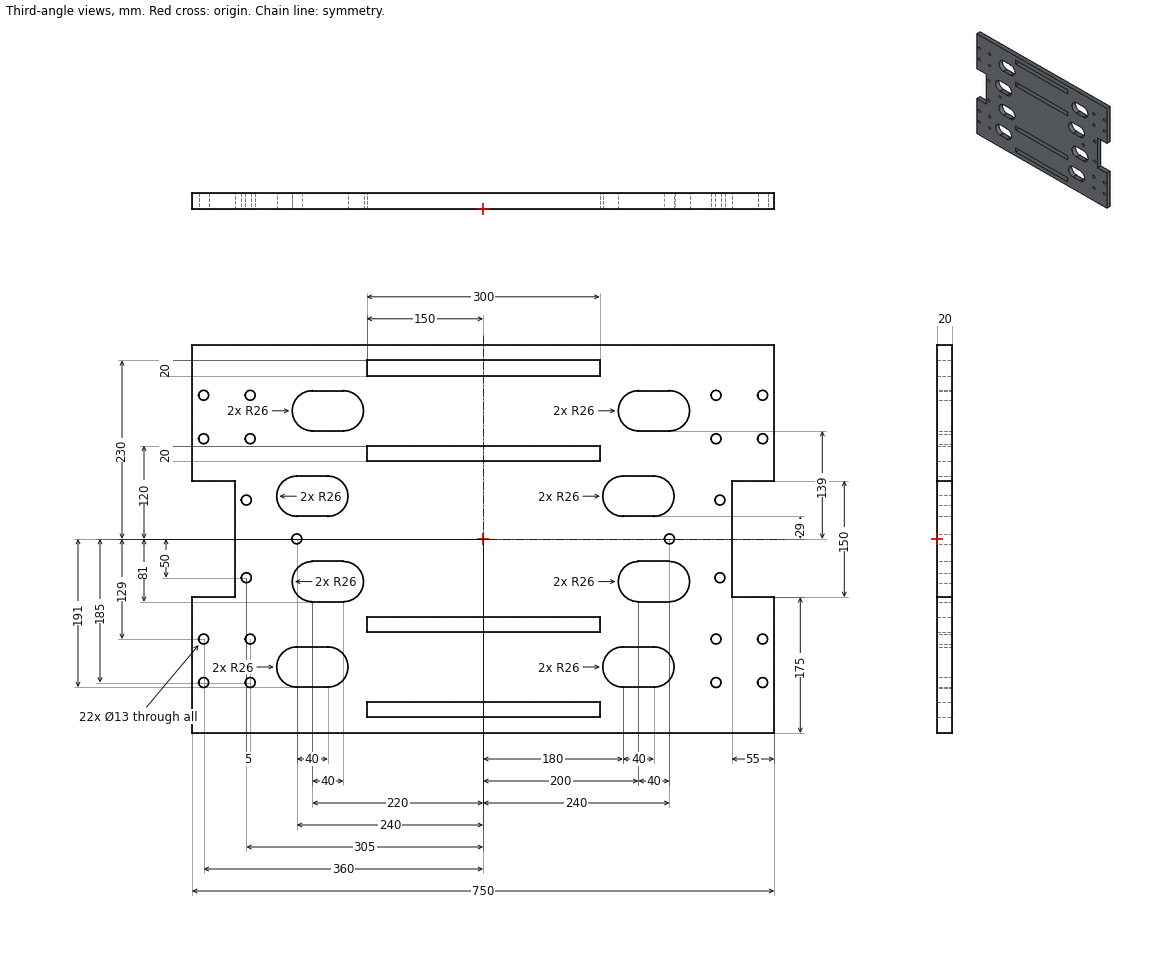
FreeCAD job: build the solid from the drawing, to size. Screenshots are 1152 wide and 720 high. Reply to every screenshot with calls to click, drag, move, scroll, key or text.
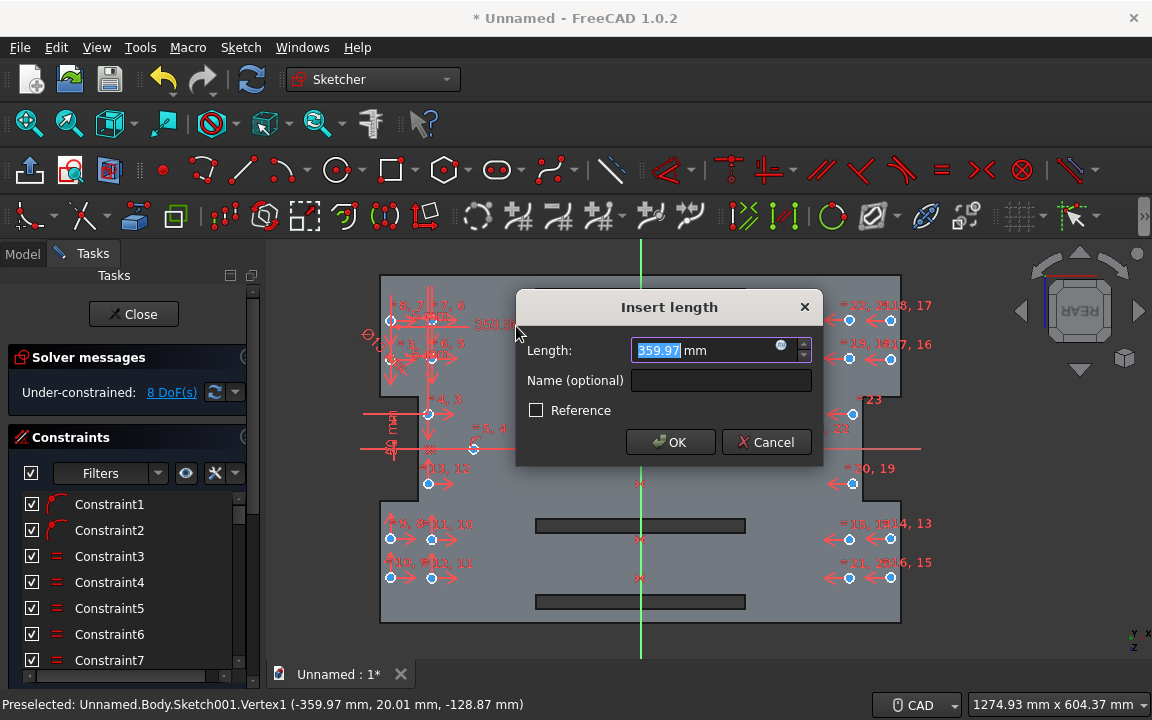
text(360)
key(Return)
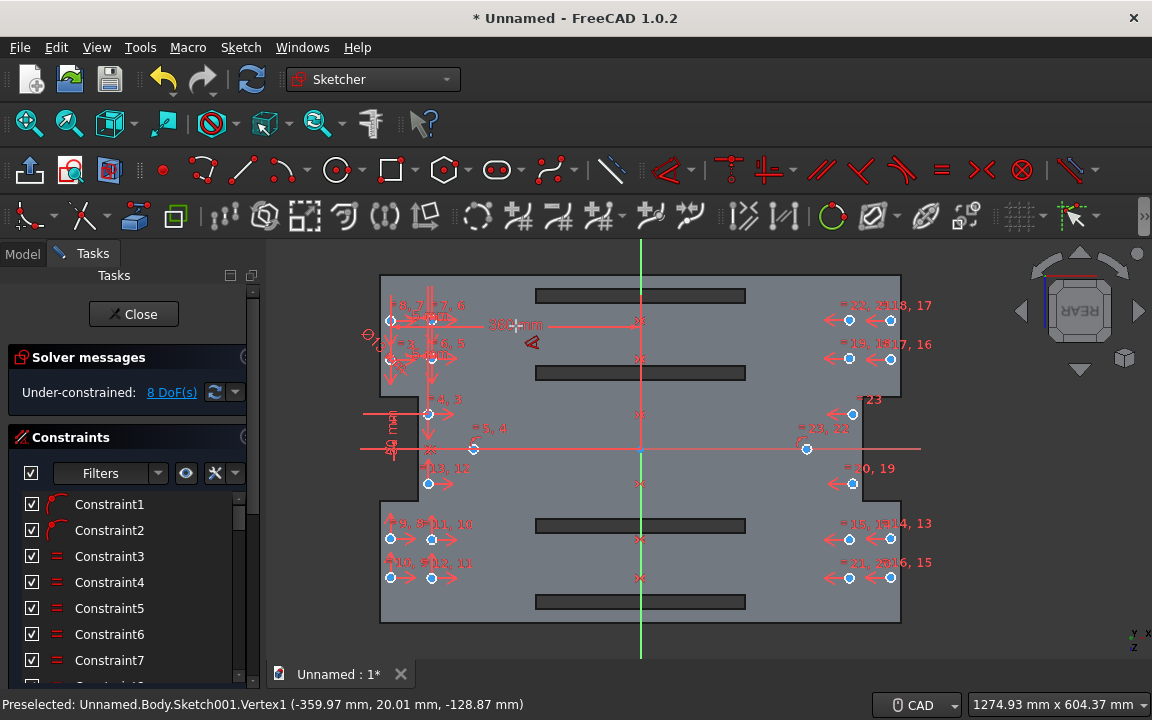
click(391, 360)
click(357, 404)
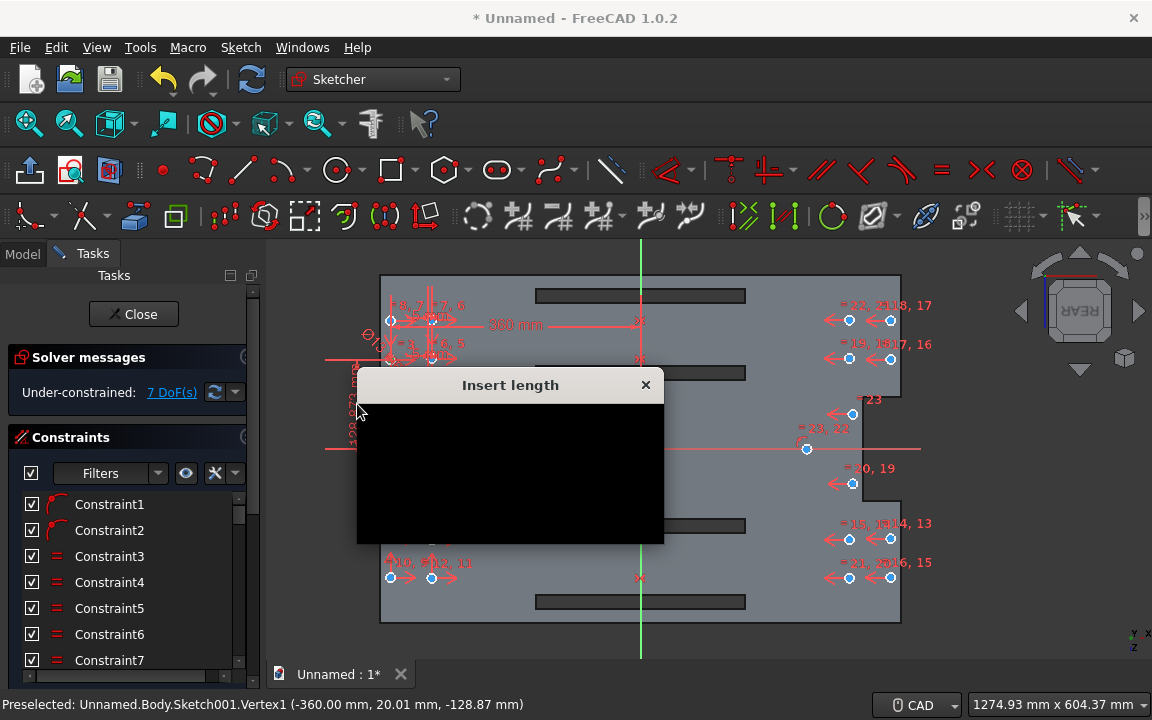
text(129)
key(Return)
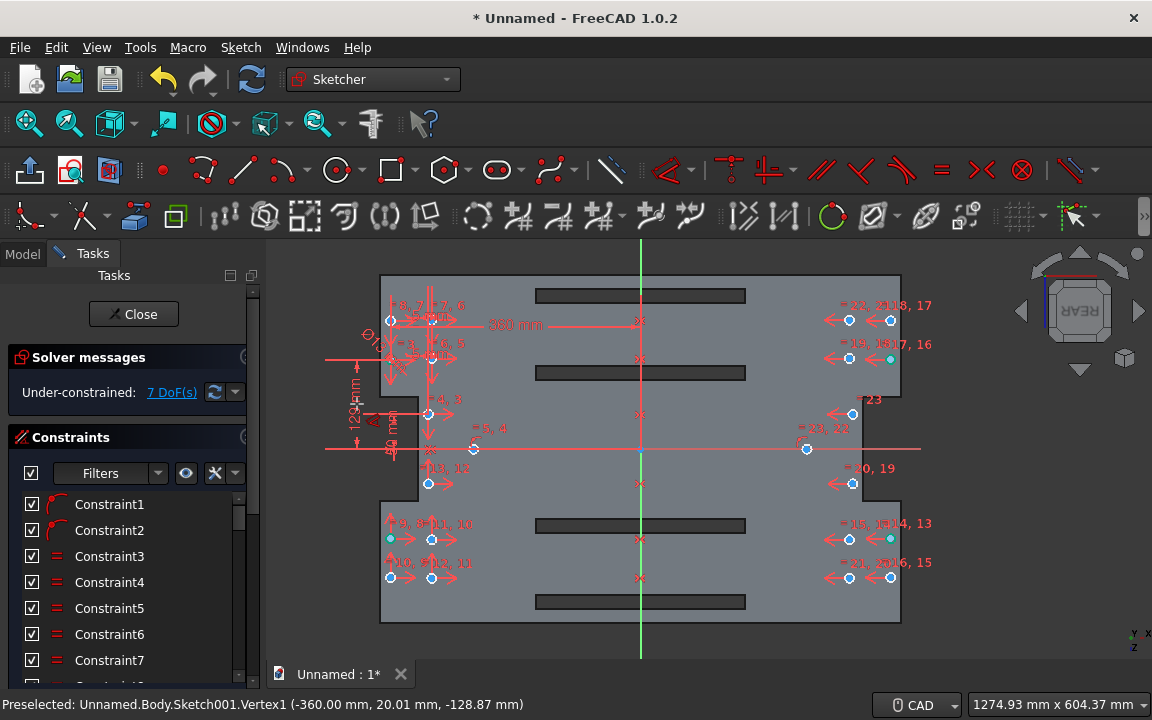
click(428, 414)
click(535, 380)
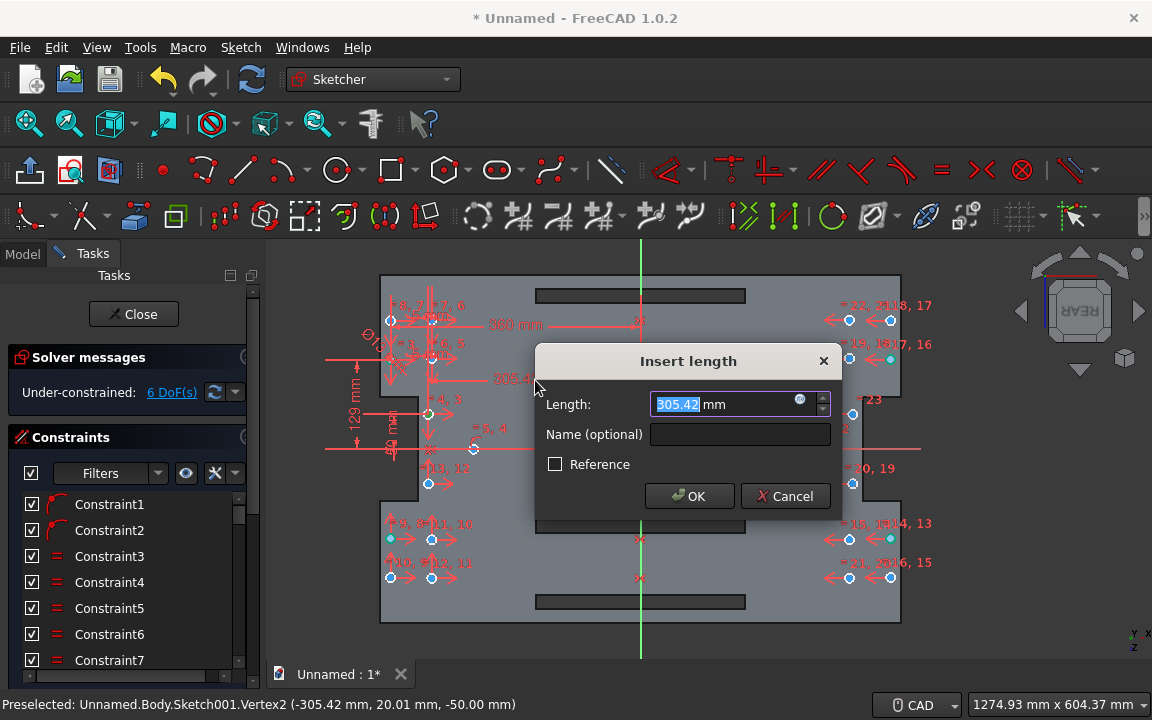
text(305)
key(Return)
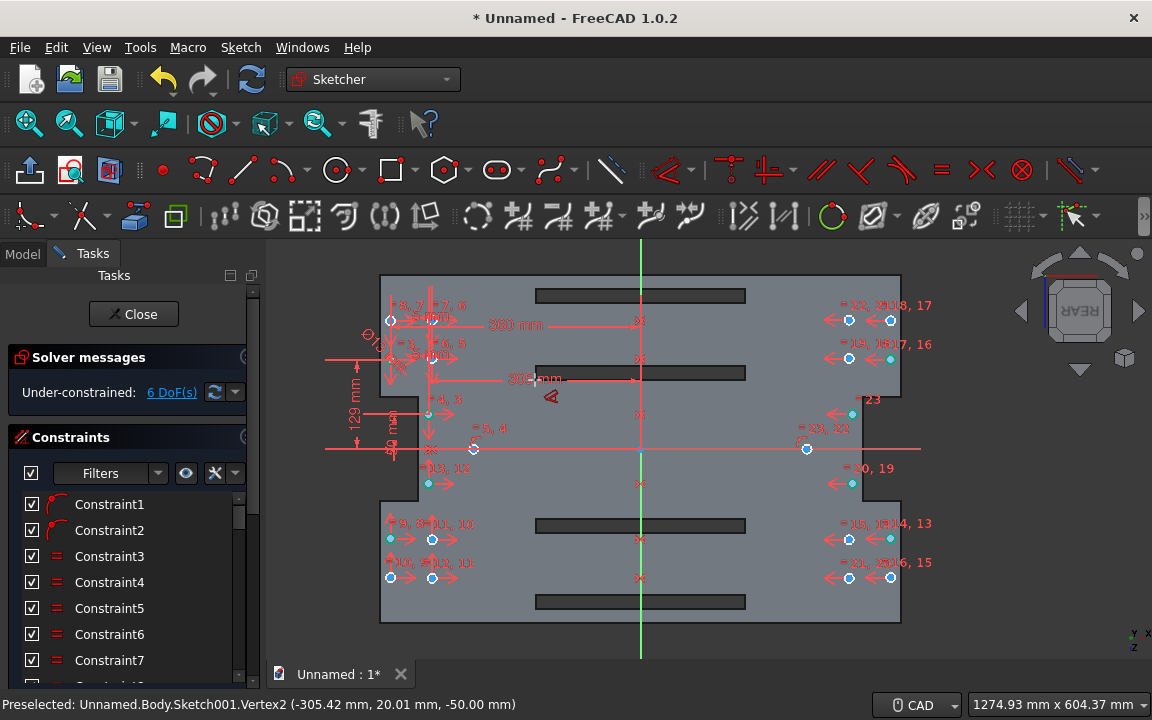
click(474, 449)
click(557, 483)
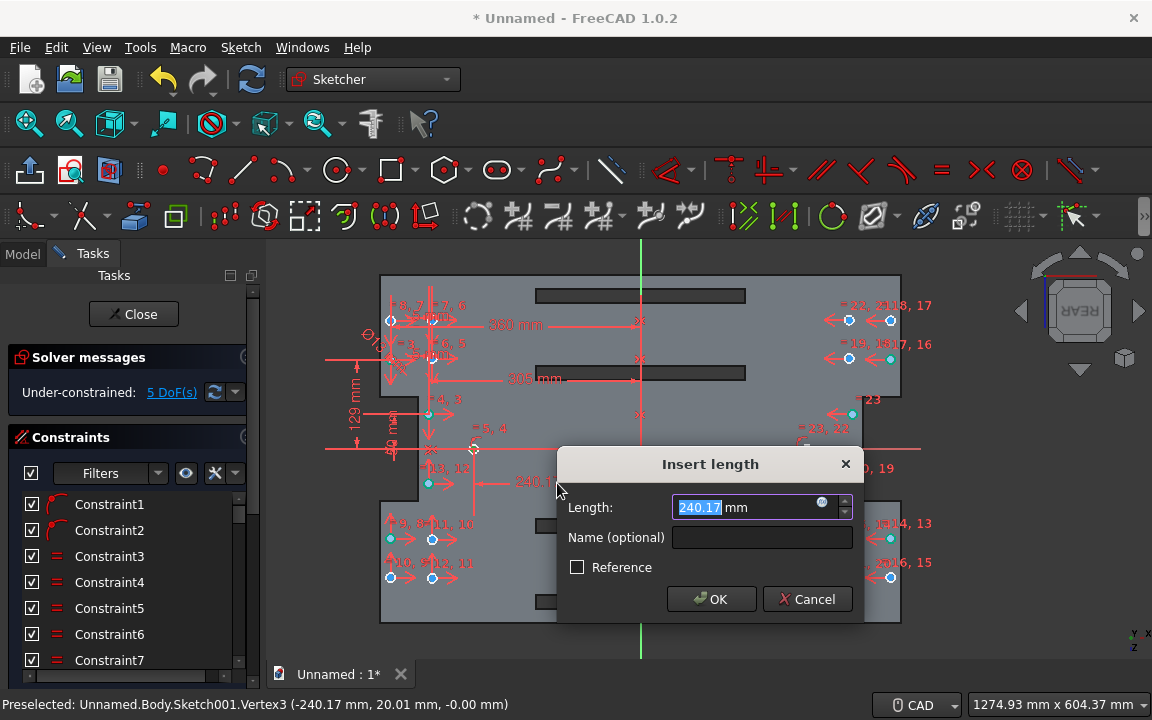
text(240)
key(Return)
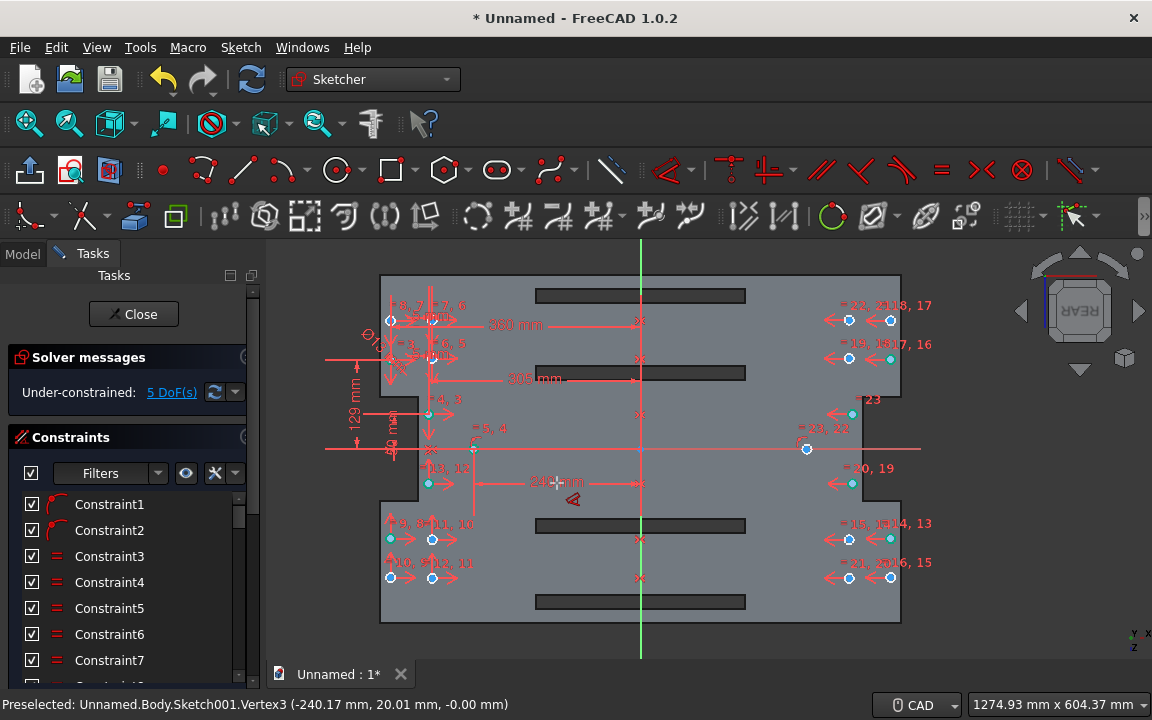
click(432, 359)
click(398, 383)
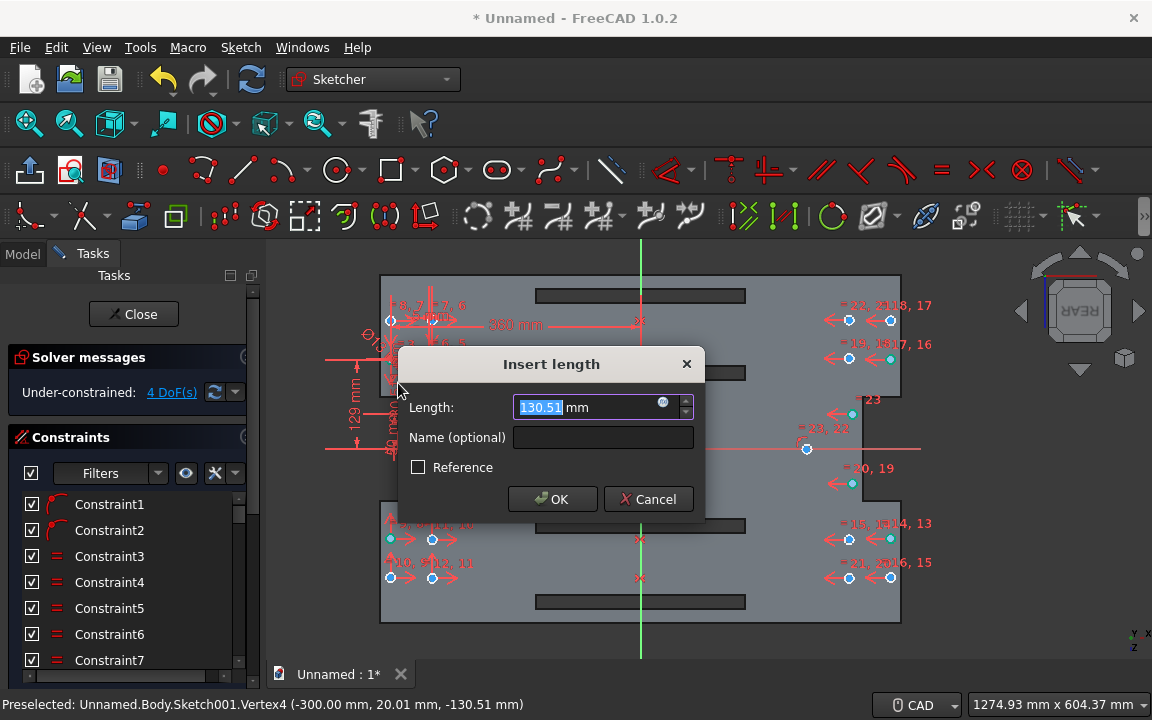
text(129)
key(Return)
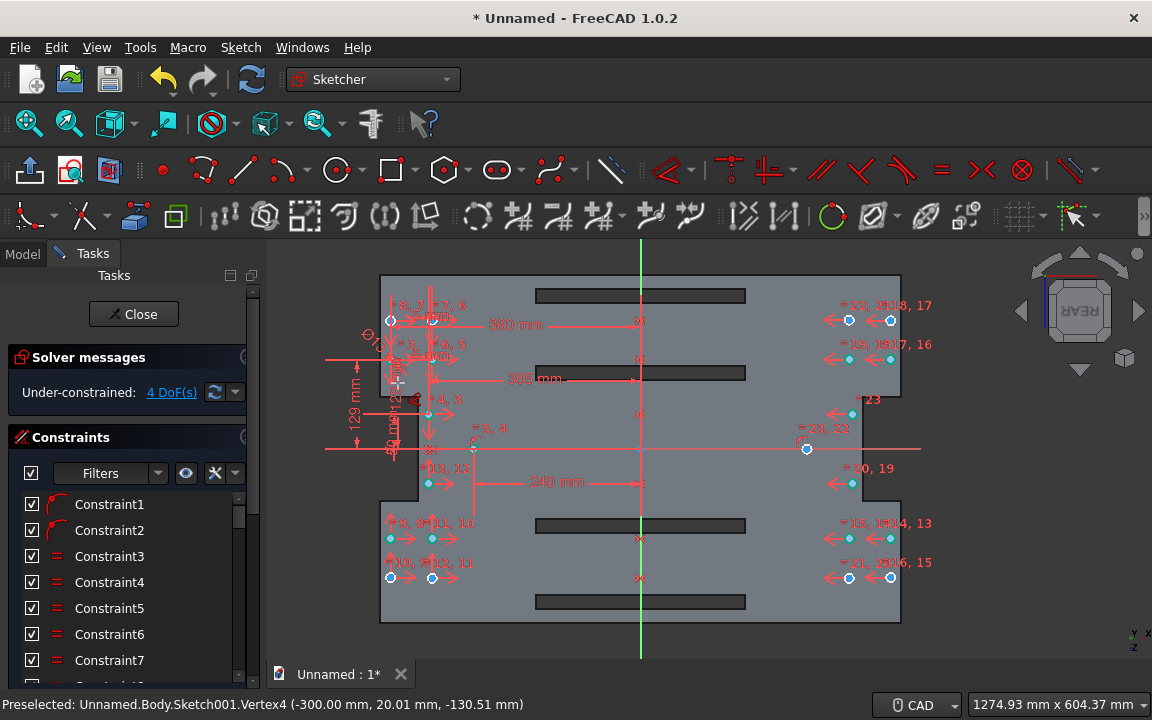
click(432, 320)
click(675, 385)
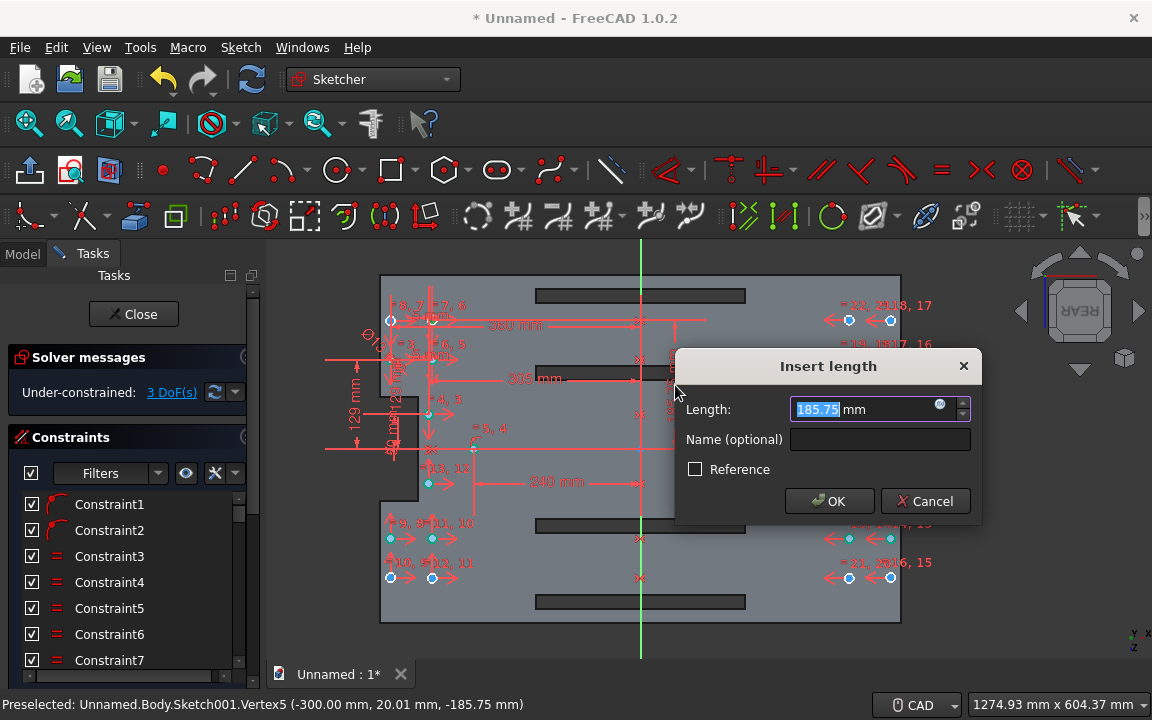
text(185)
key(Return)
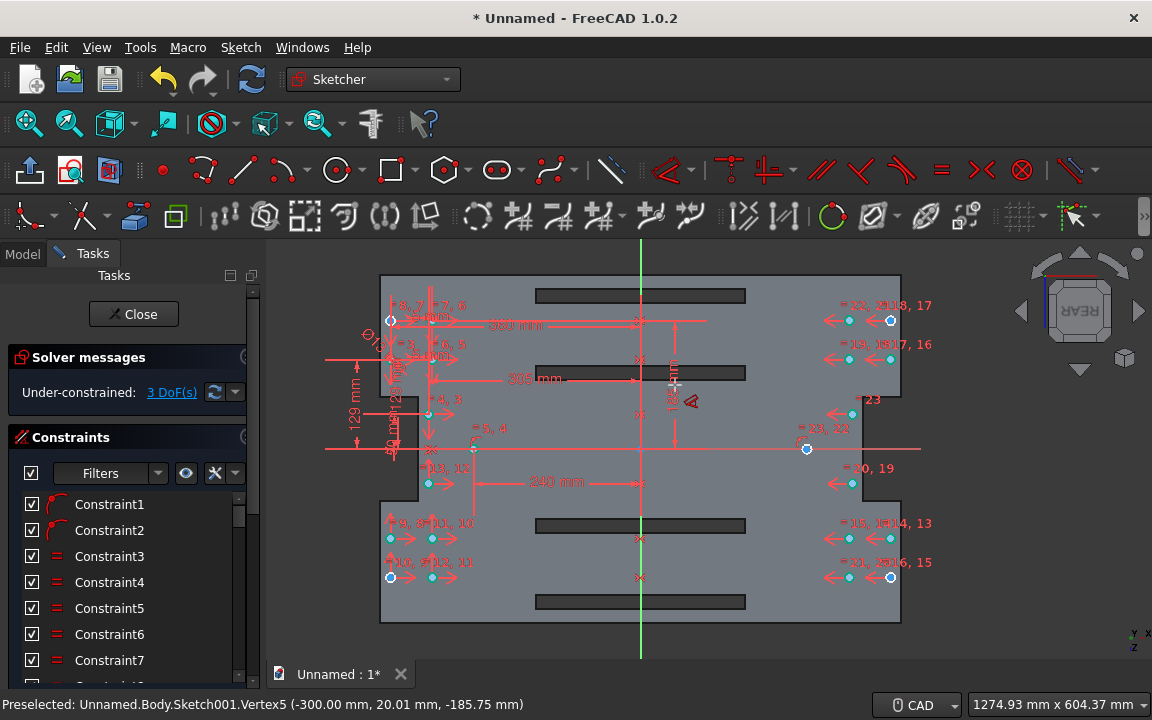
click(391, 321)
click(516, 287)